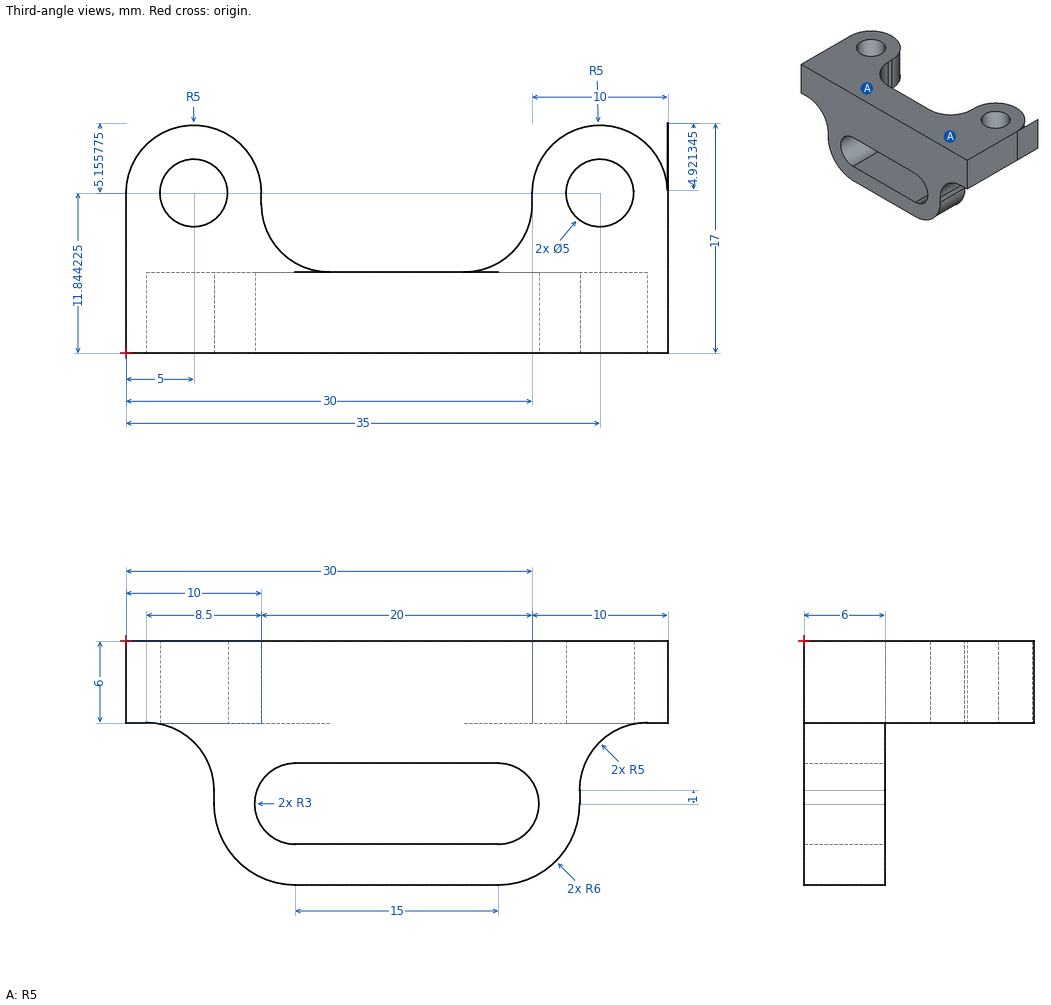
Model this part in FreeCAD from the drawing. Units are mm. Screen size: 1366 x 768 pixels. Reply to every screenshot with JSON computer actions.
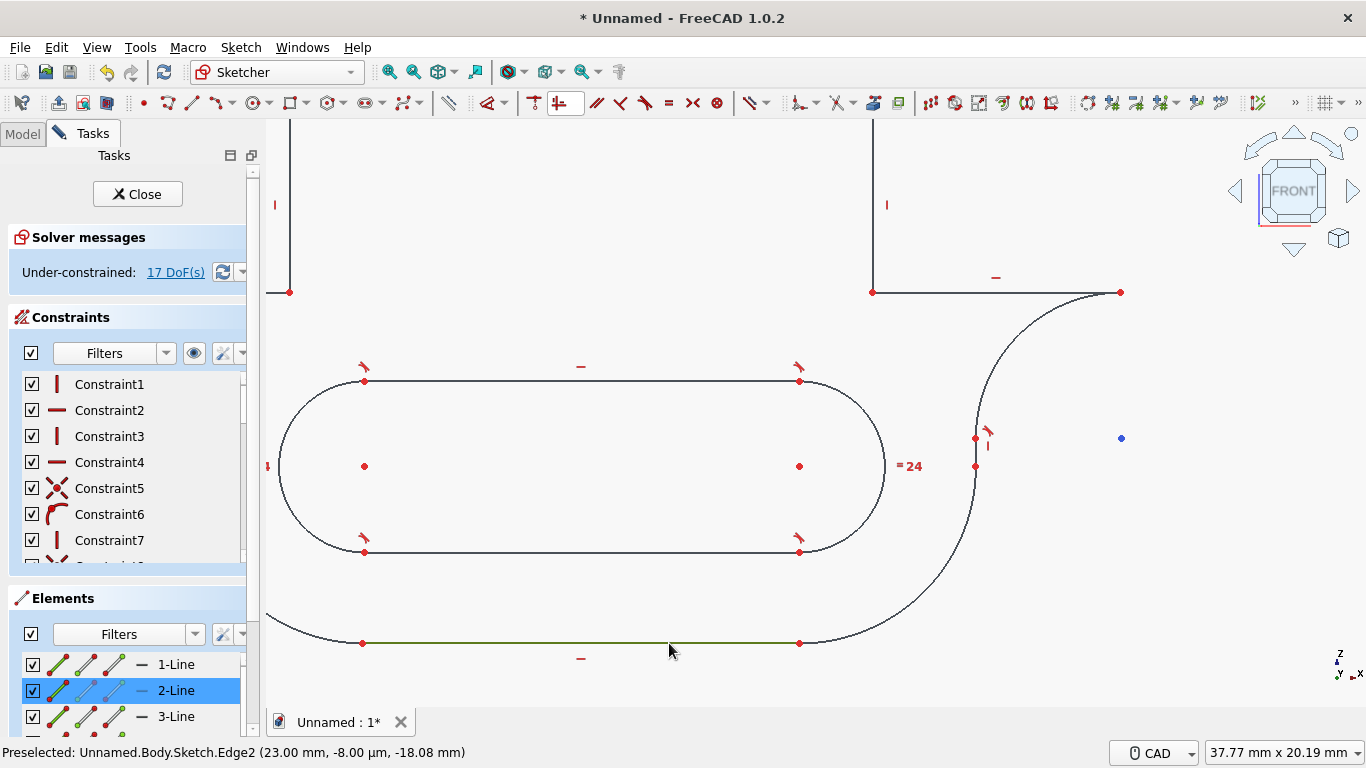
{"action": "left_click", "coordinate": [880, 624]}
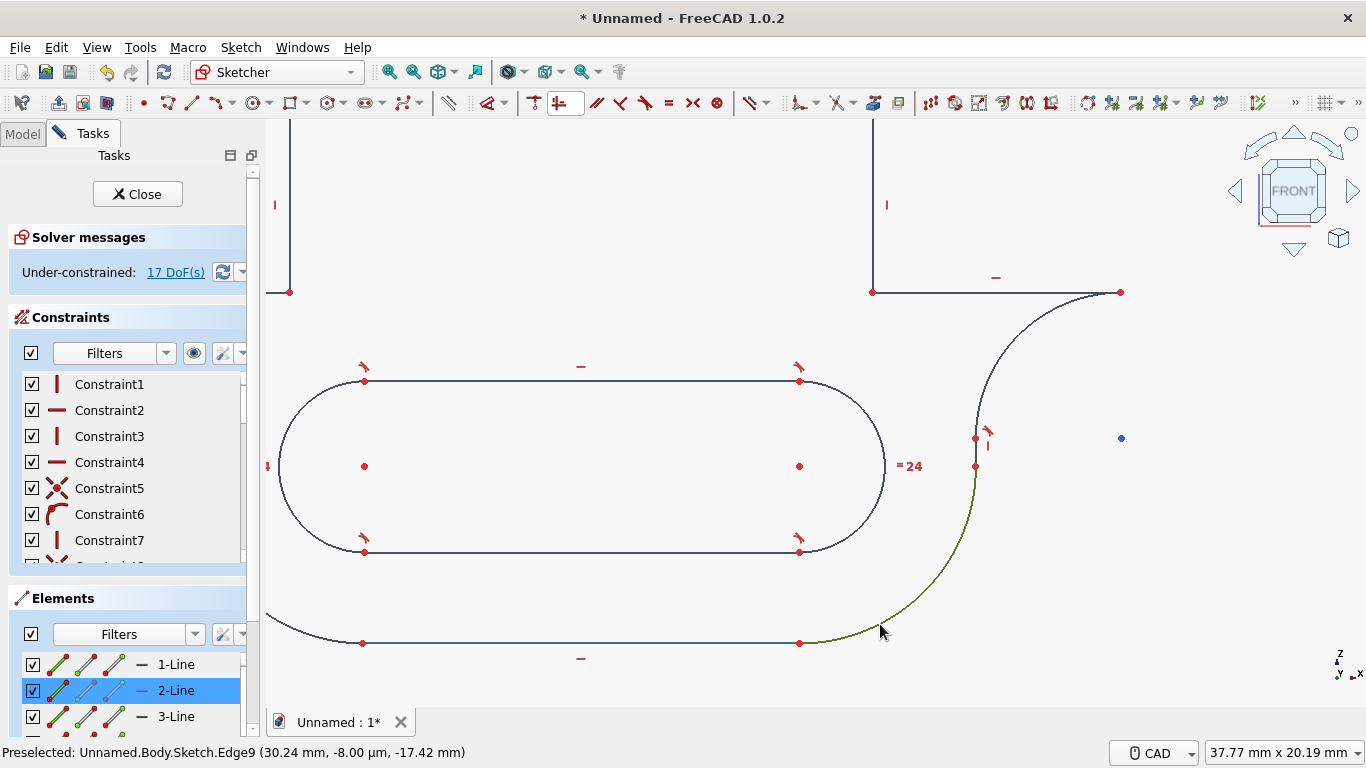
{"action": "key", "text": "t"}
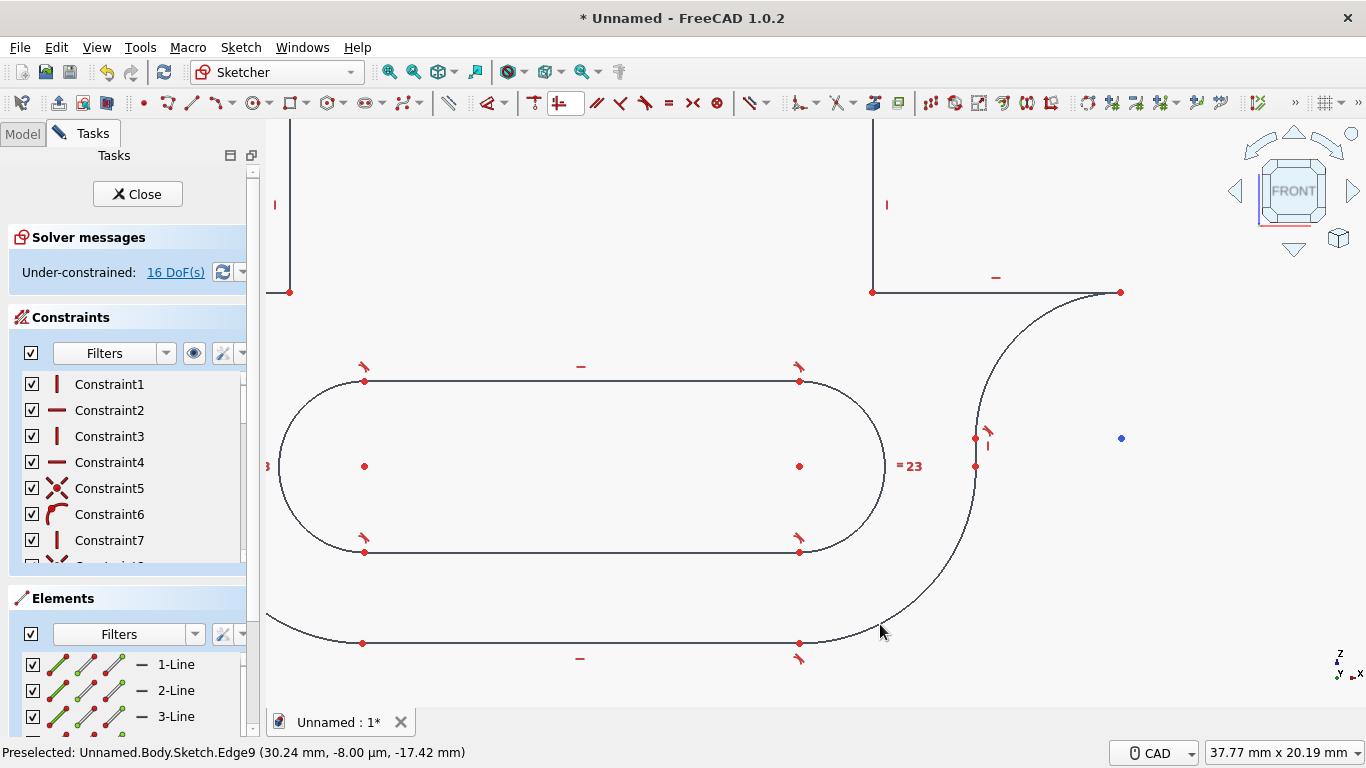
{"action": "left_click", "coordinate": [668, 643]}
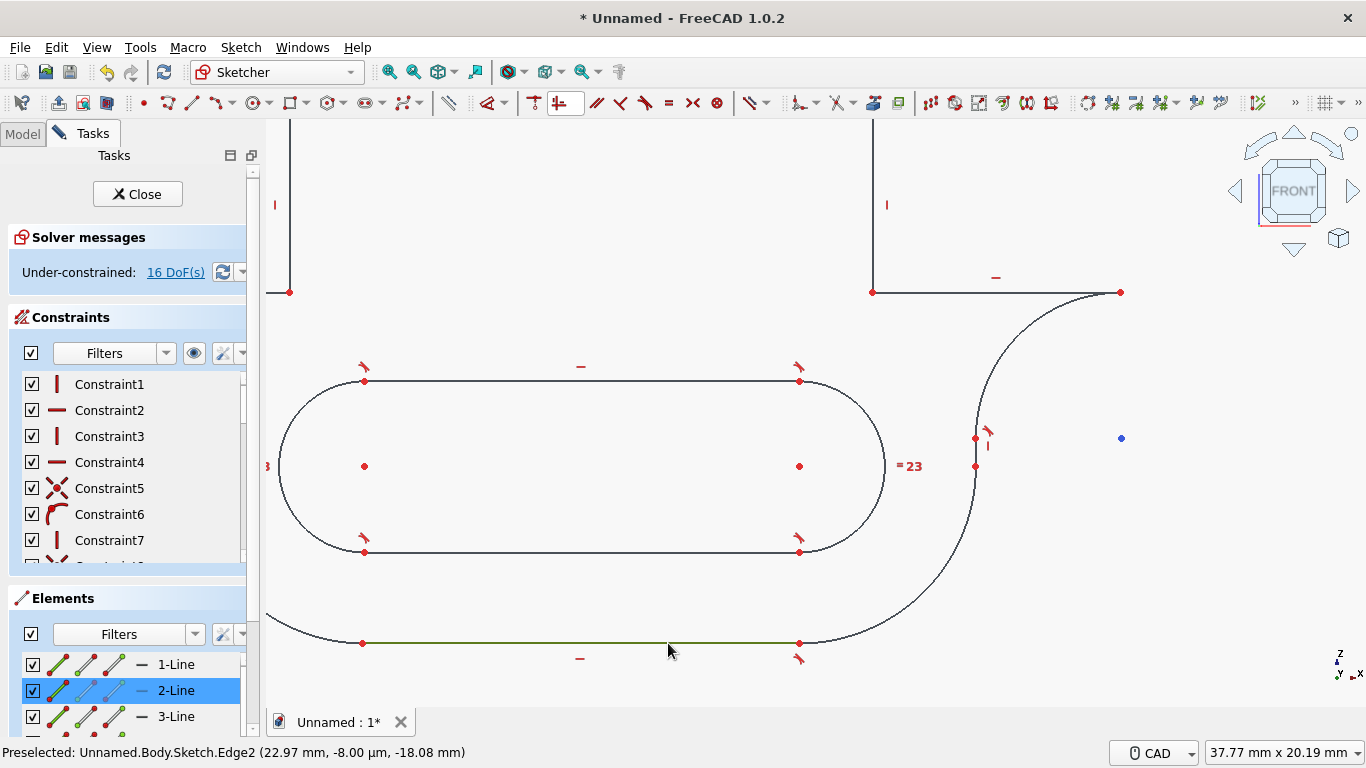
{"action": "left_click", "coordinate": [309, 634]}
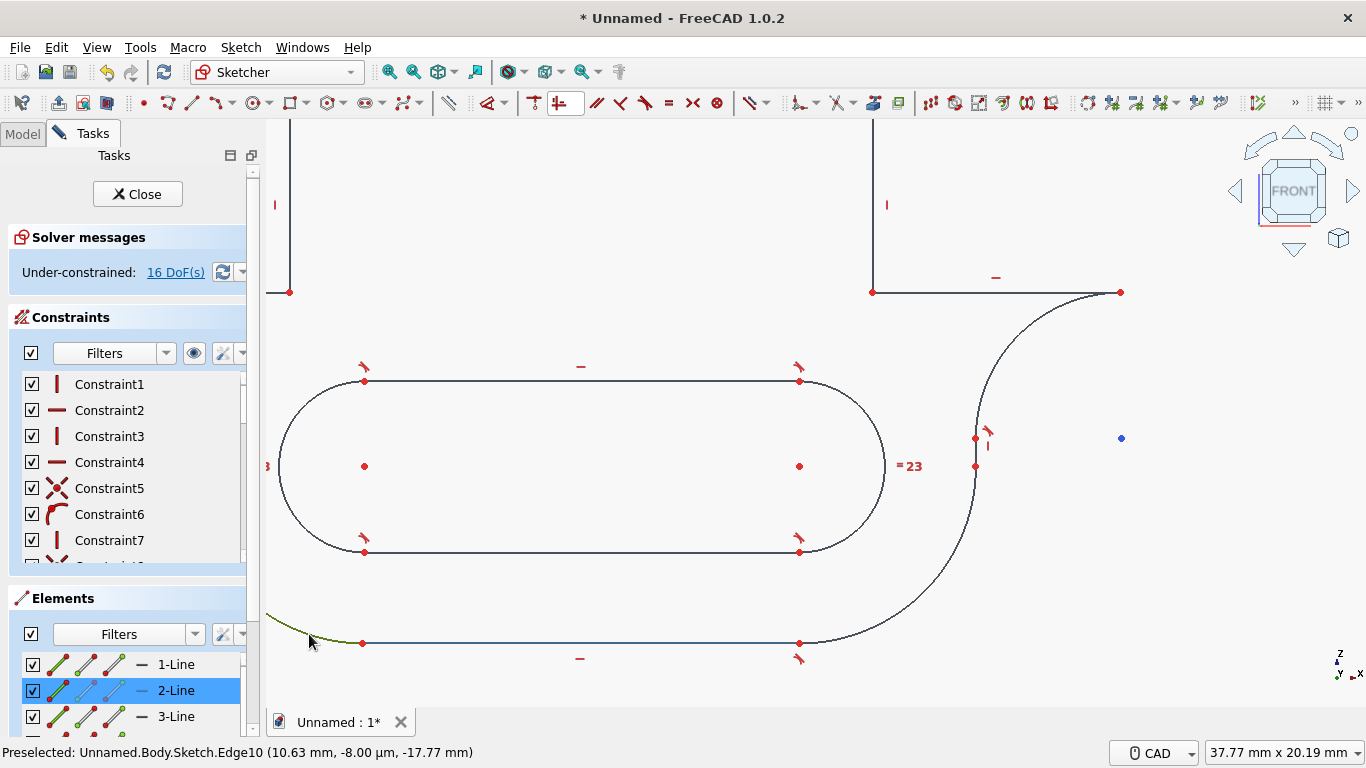
{"action": "left_click", "coordinate": [646, 104]}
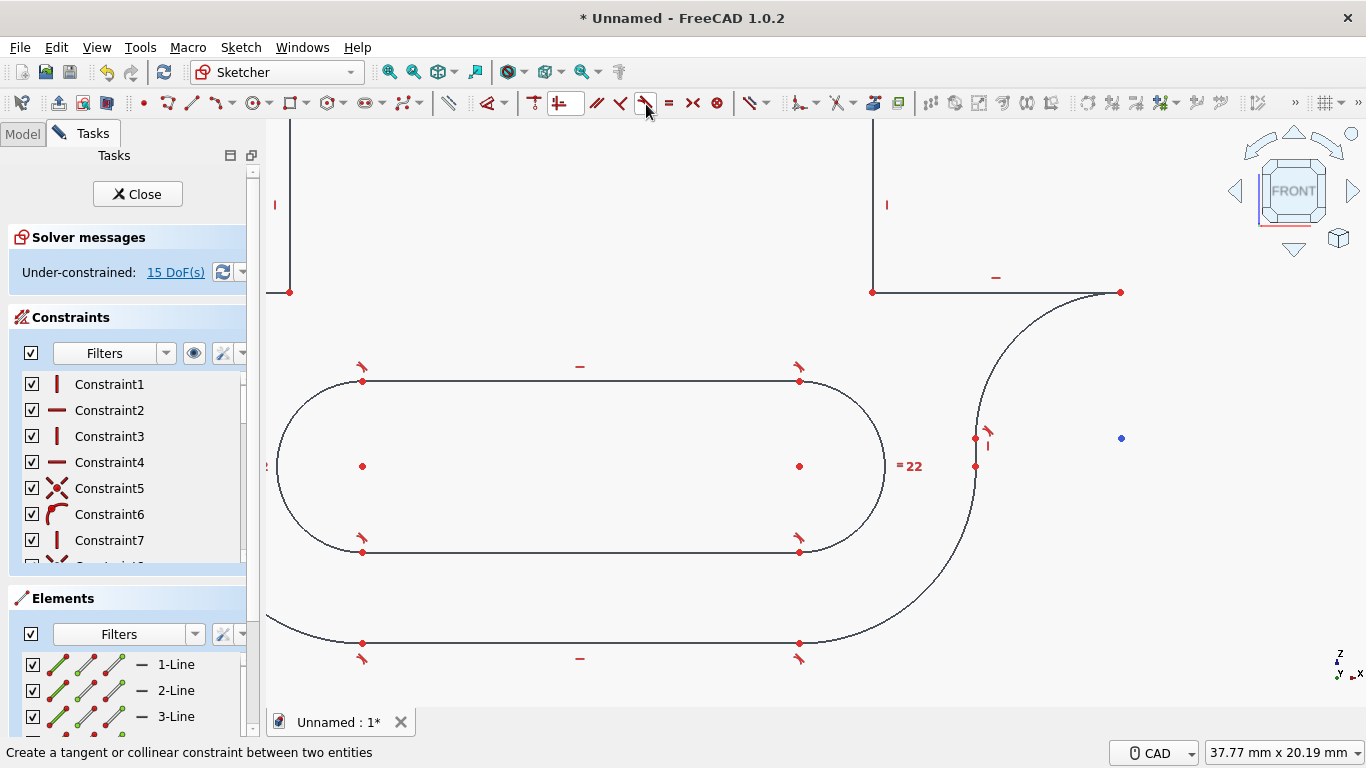
{"action": "scroll", "coordinate": [976, 454], "scroll_direction": "down", "scroll_amount": 3}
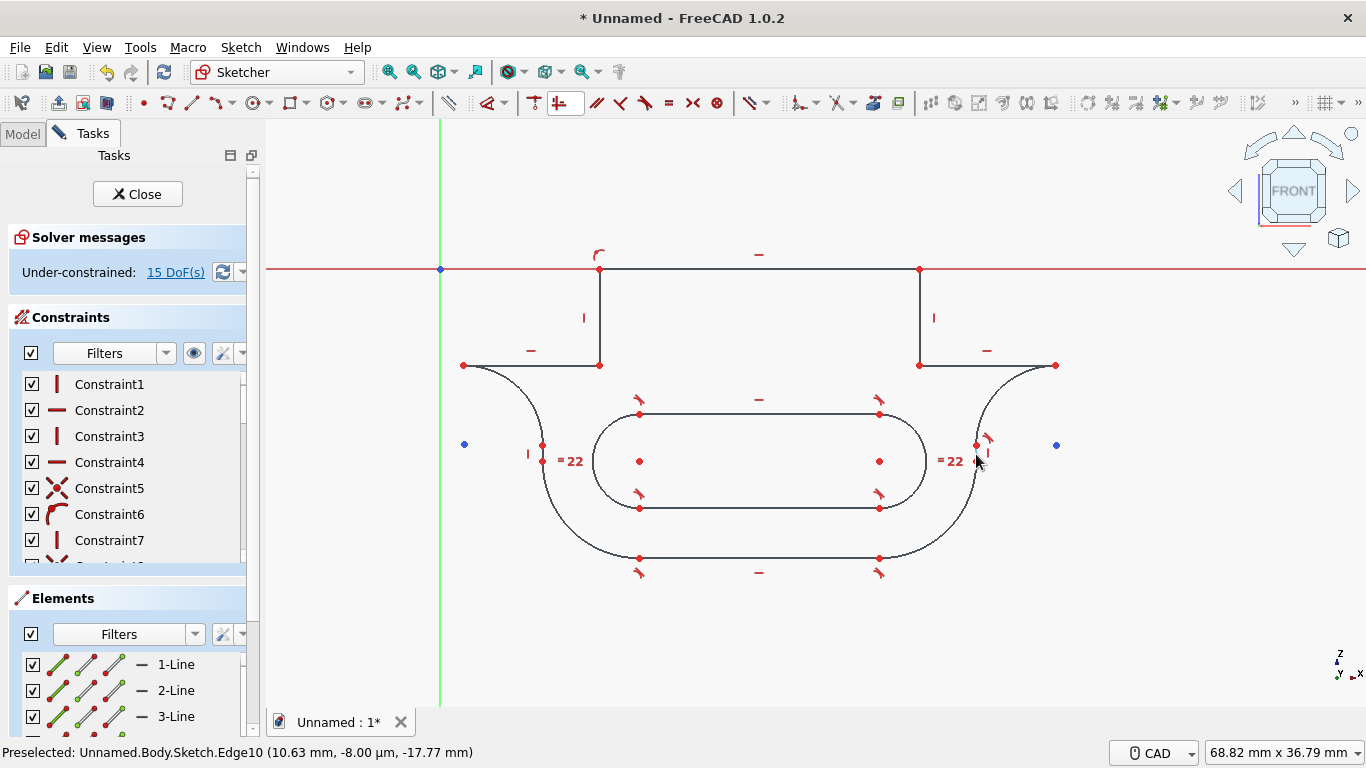
{"action": "scroll", "coordinate": [543, 455], "scroll_direction": "up", "scroll_amount": 4}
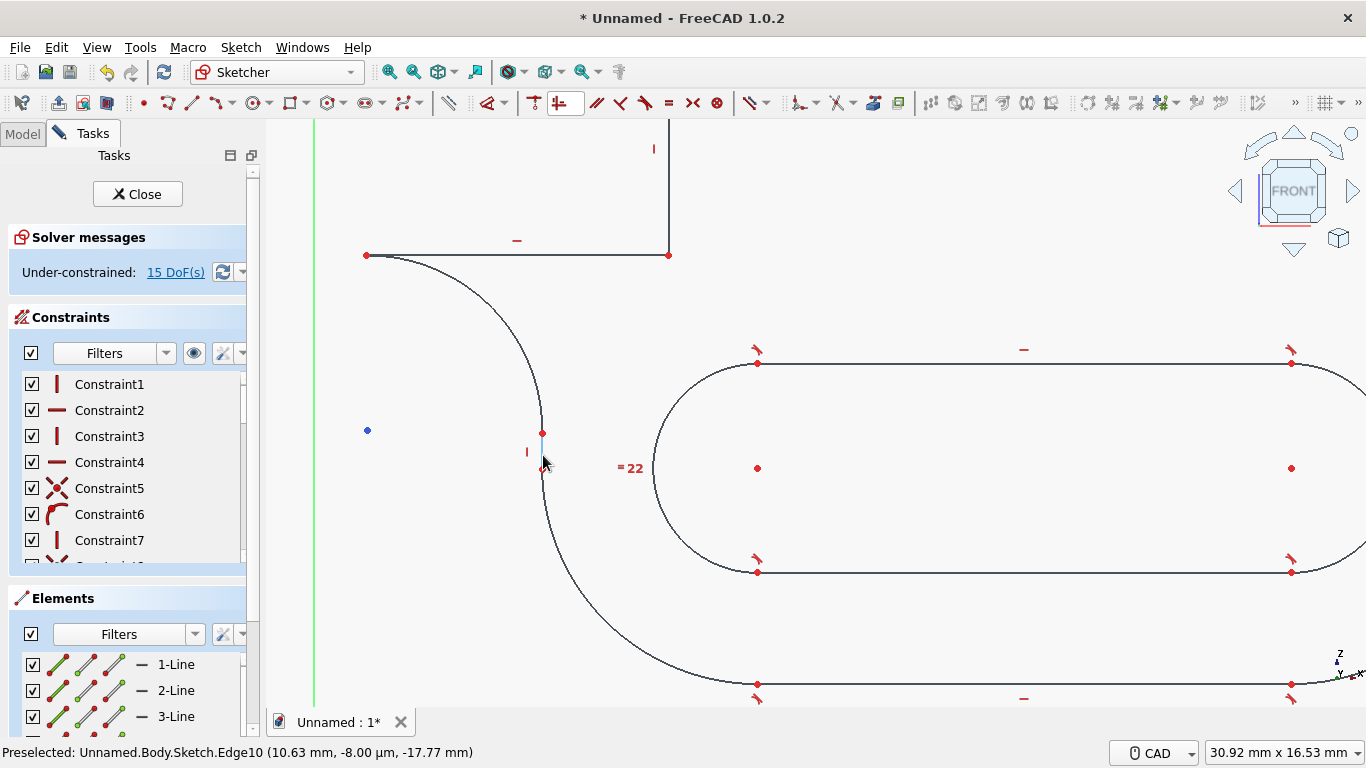
{"action": "left_click", "coordinate": [542, 455]}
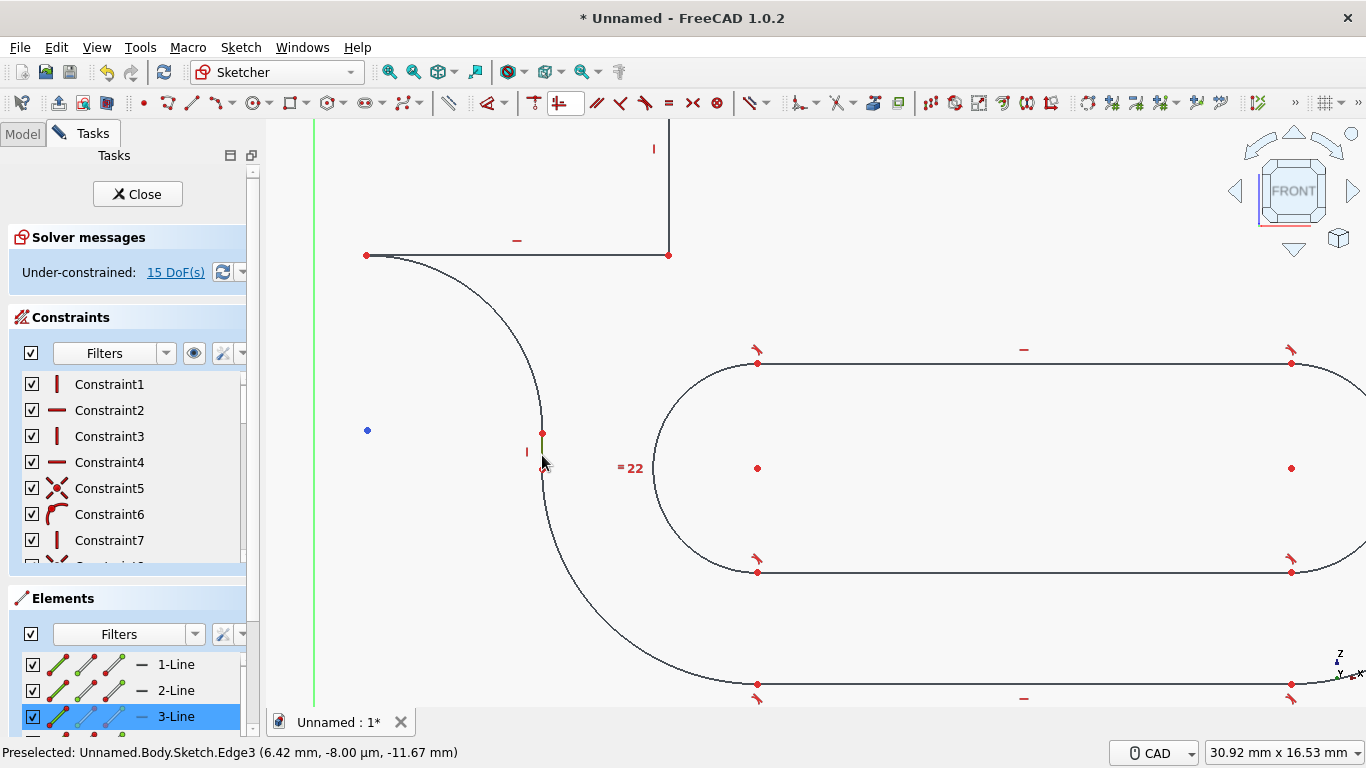
{"action": "left_click", "coordinate": [566, 567]}